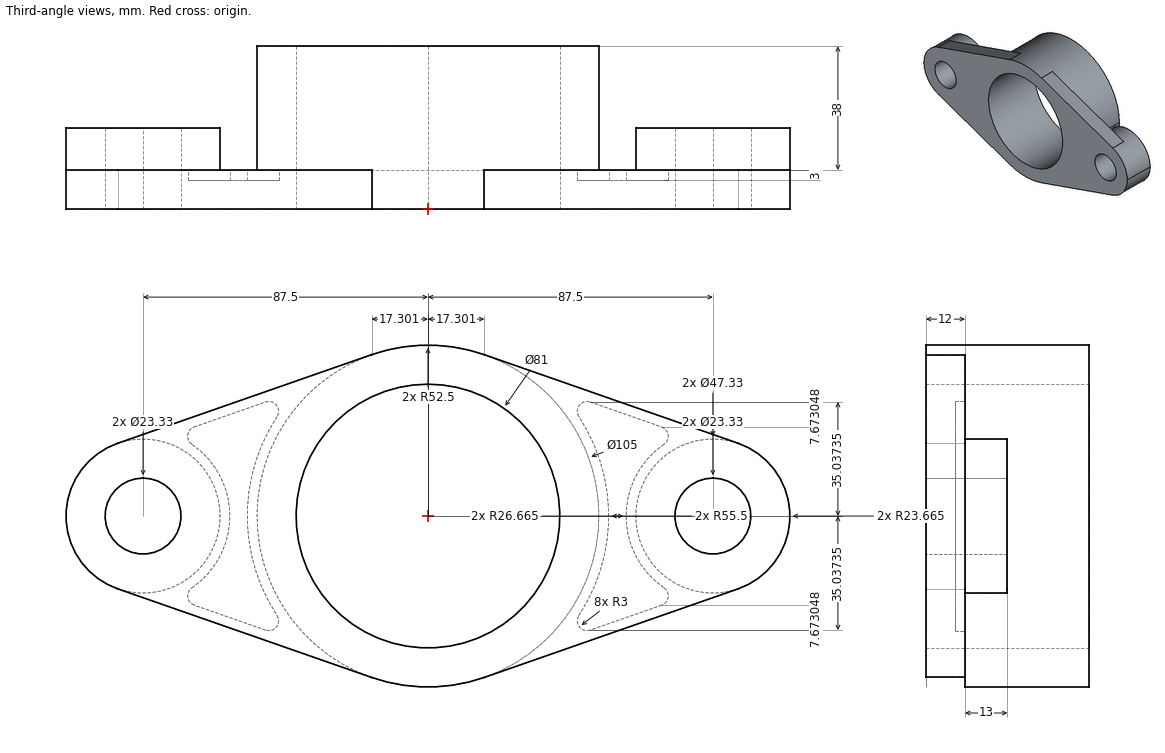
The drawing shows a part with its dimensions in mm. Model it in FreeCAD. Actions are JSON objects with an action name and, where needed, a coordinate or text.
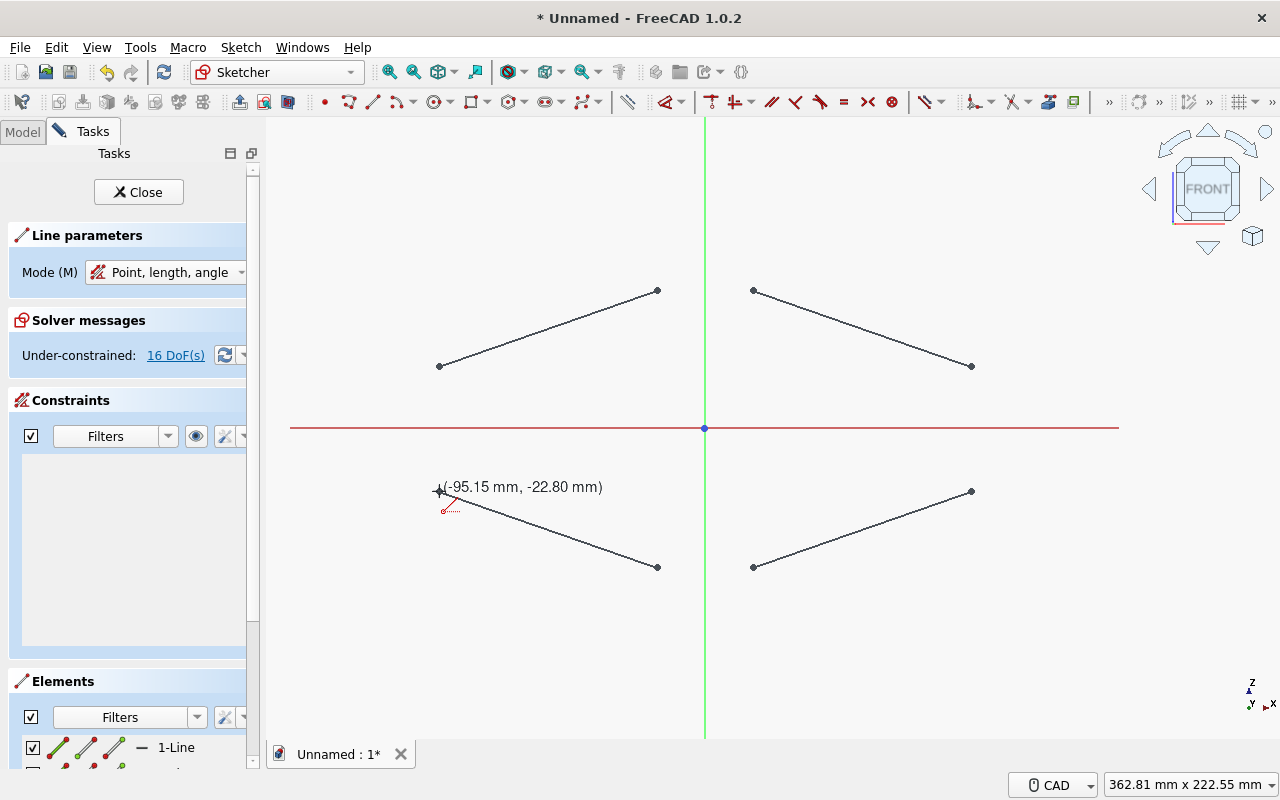
{"action": "key", "text": "g 3 a"}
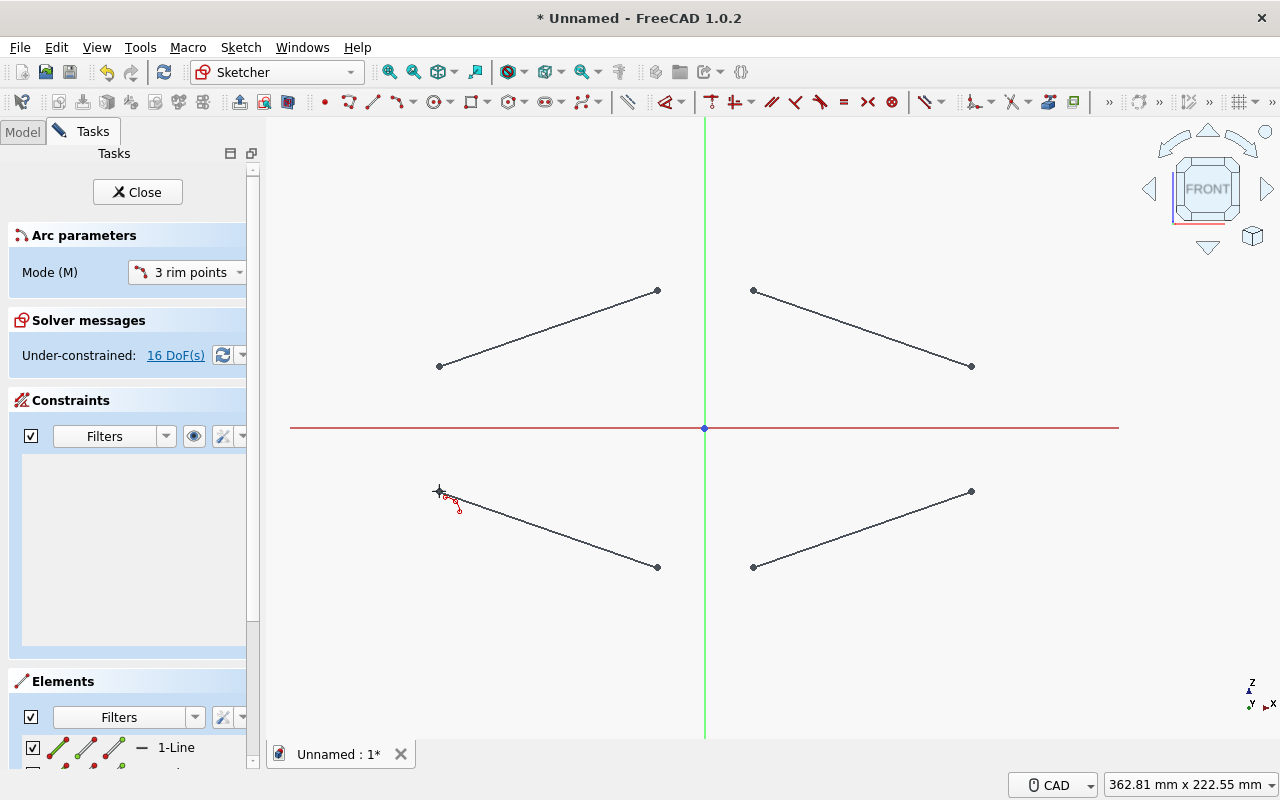
{"action": "left_click", "coordinate": [657, 291]}
{"action": "left_click", "coordinate": [753, 291]}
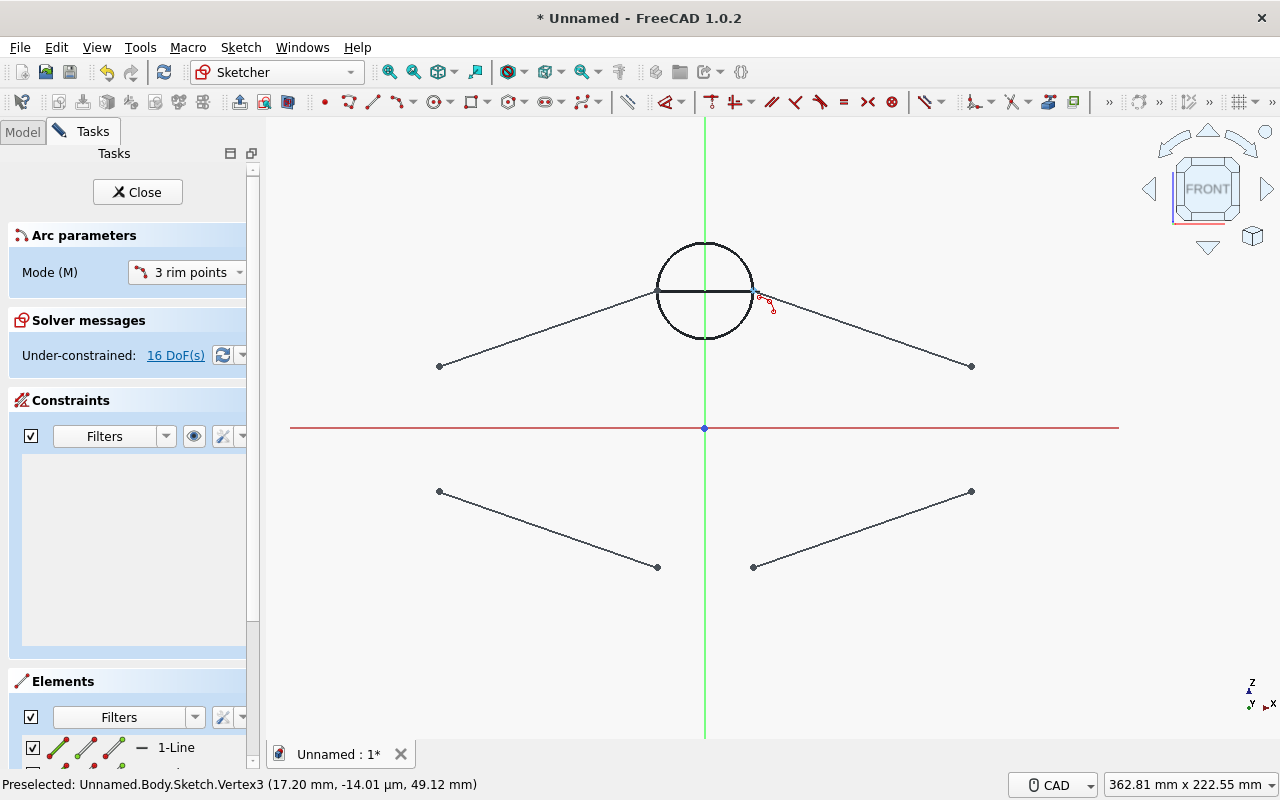
{"action": "scroll", "coordinate": [715, 282], "scroll_direction": "up", "scroll_amount": 4}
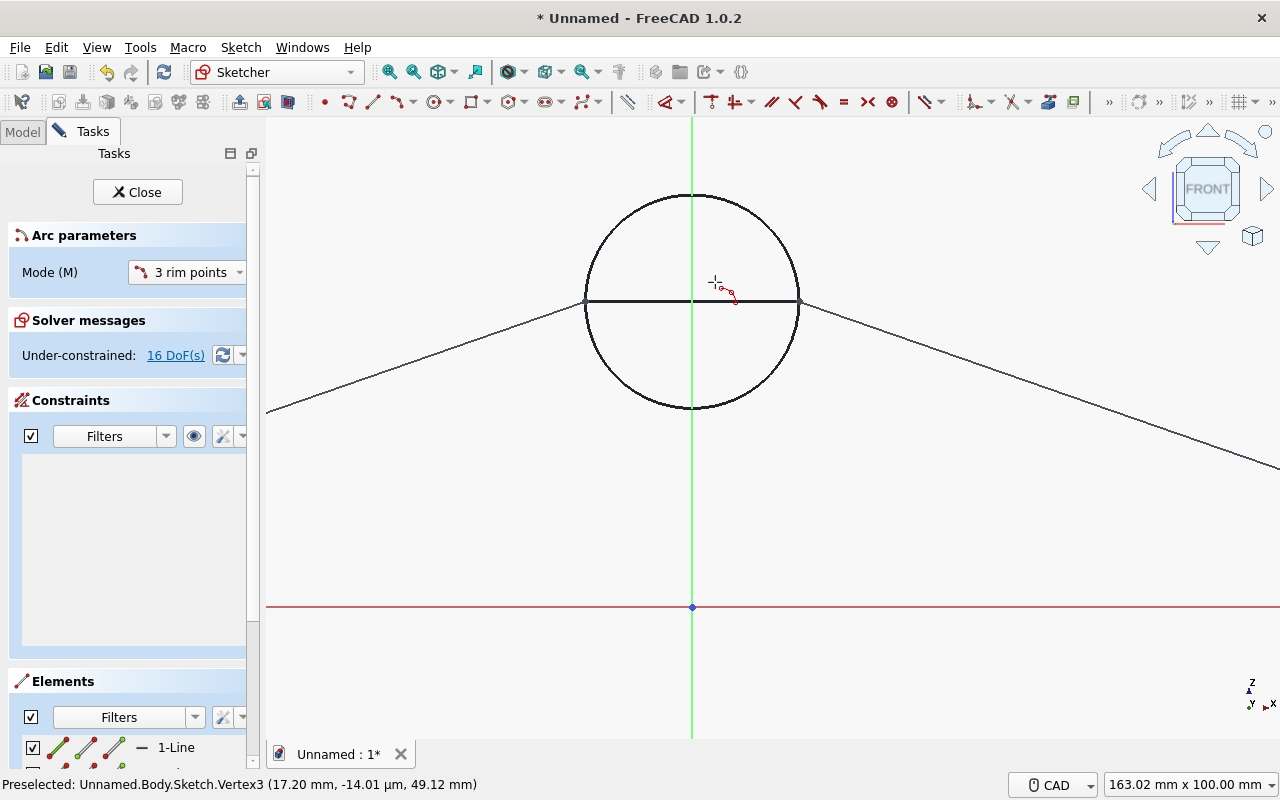
{"action": "left_click", "coordinate": [714, 281]}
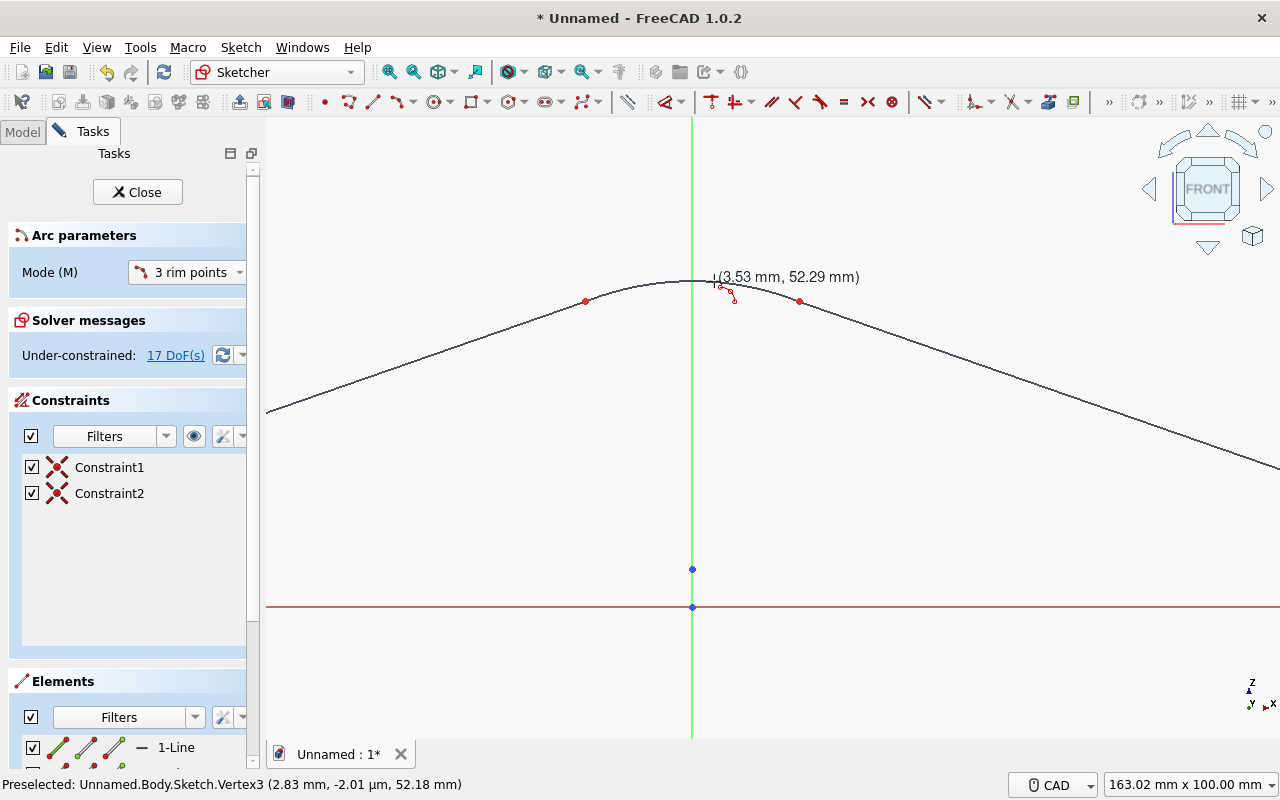
{"action": "scroll", "coordinate": [715, 282], "scroll_direction": "down", "scroll_amount": 4}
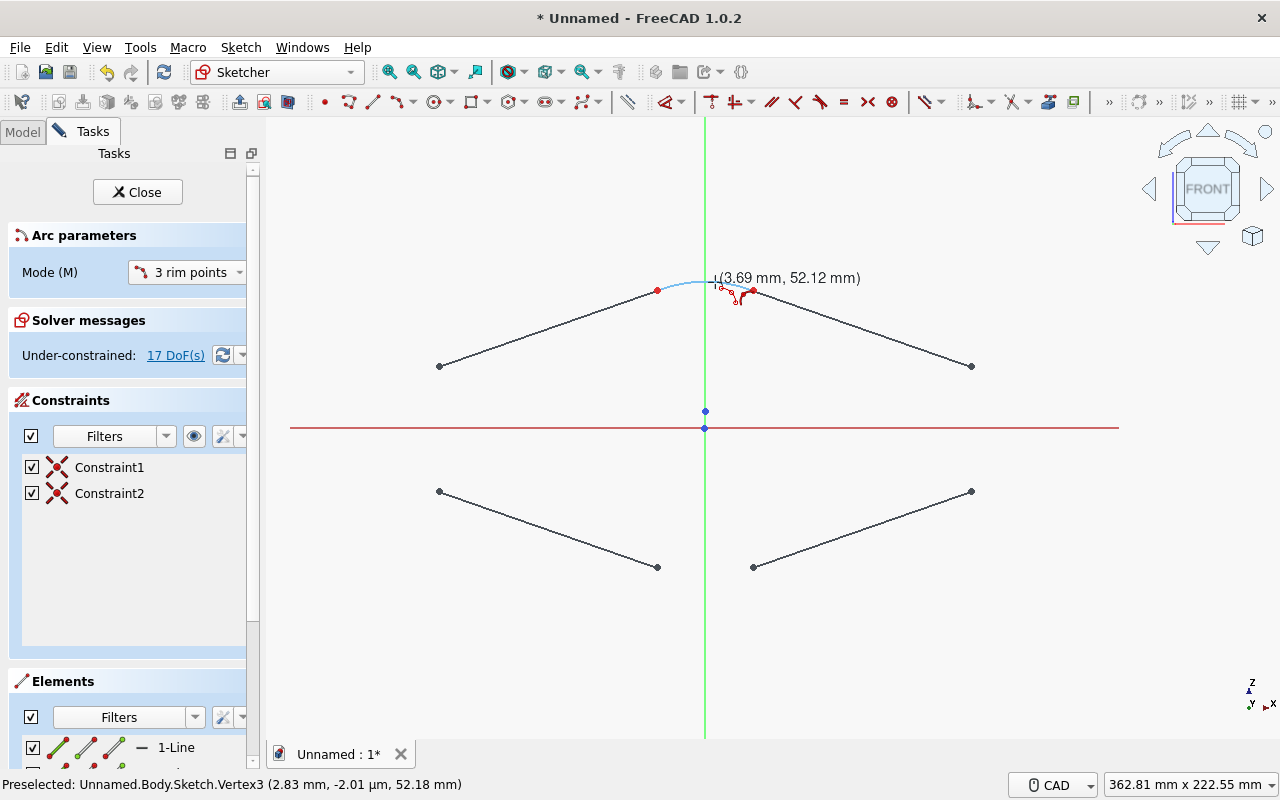
{"action": "left_click", "coordinate": [971, 367]}
{"action": "left_click", "coordinate": [971, 492]}
{"action": "left_click", "coordinate": [1014, 444]}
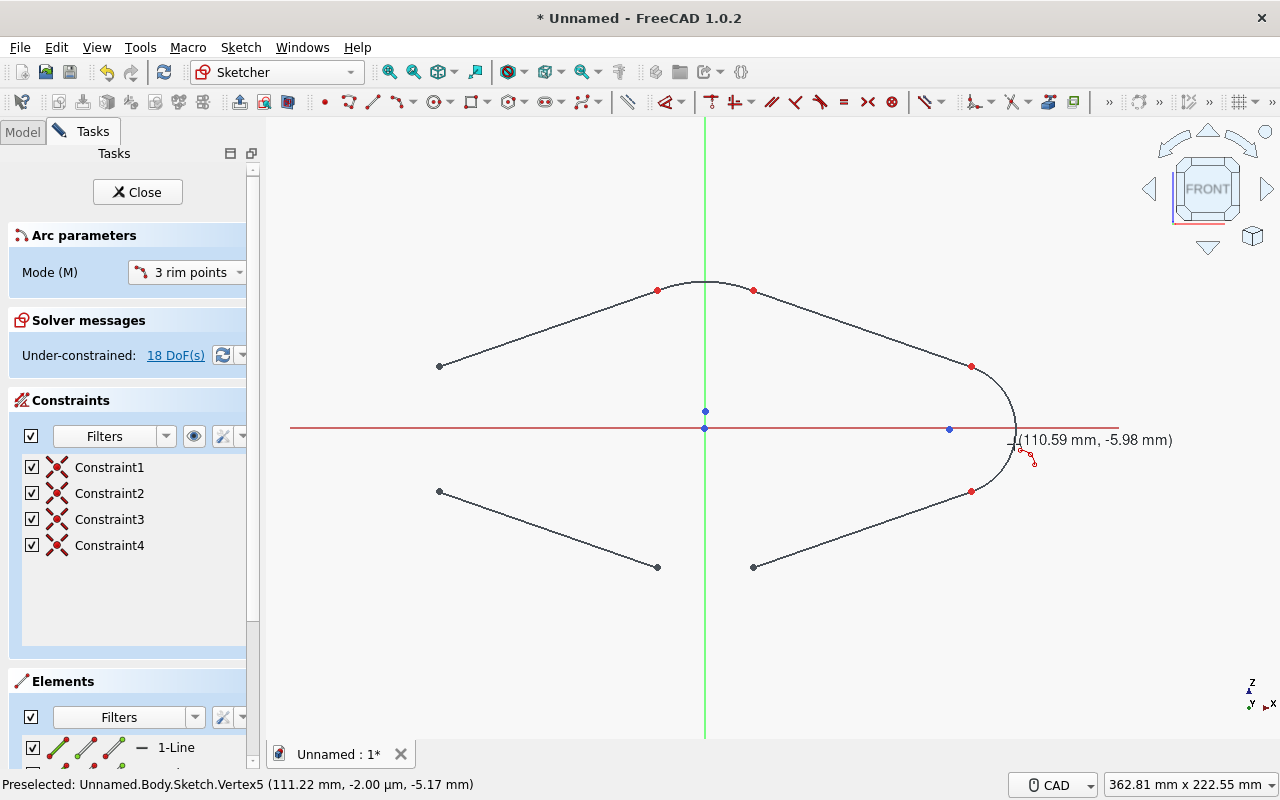
{"action": "left_click", "coordinate": [753, 568]}
{"action": "left_click", "coordinate": [657, 568]}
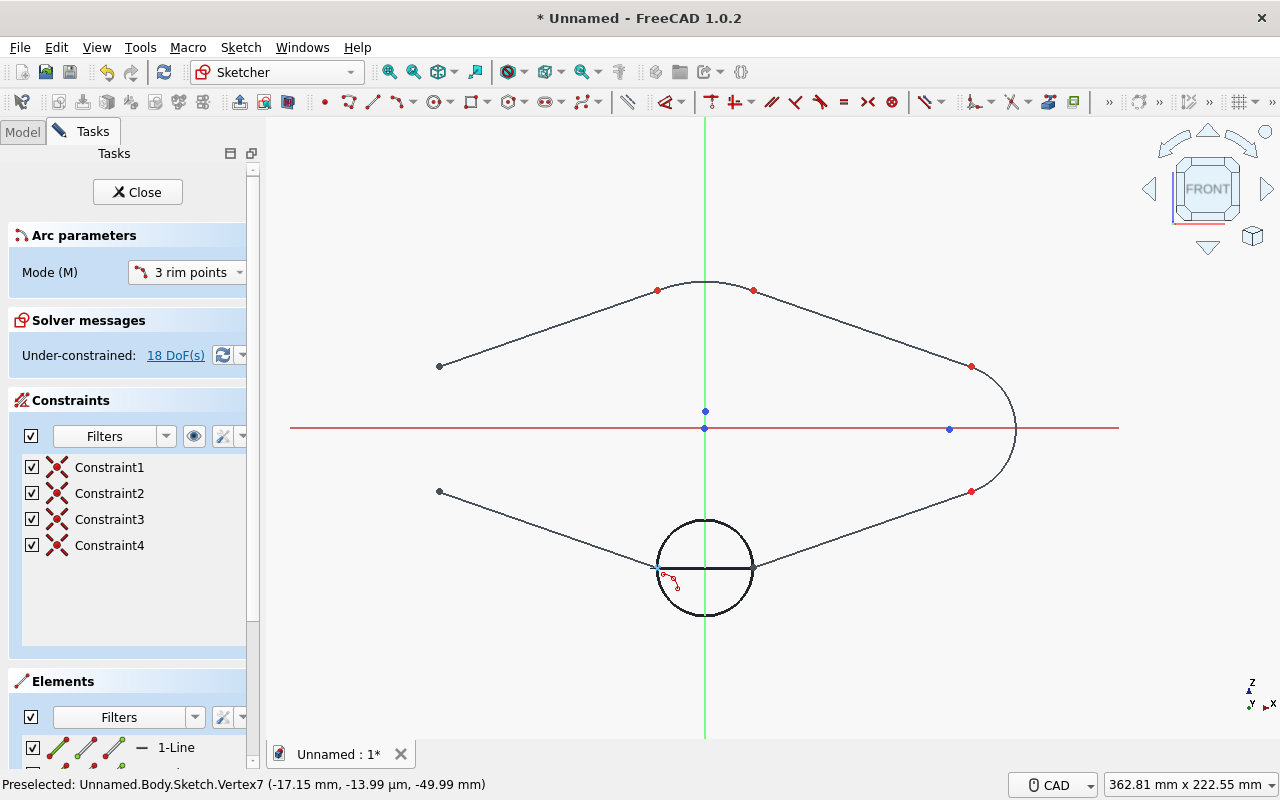
{"action": "scroll", "coordinate": [695, 575], "scroll_direction": "up", "scroll_amount": 4}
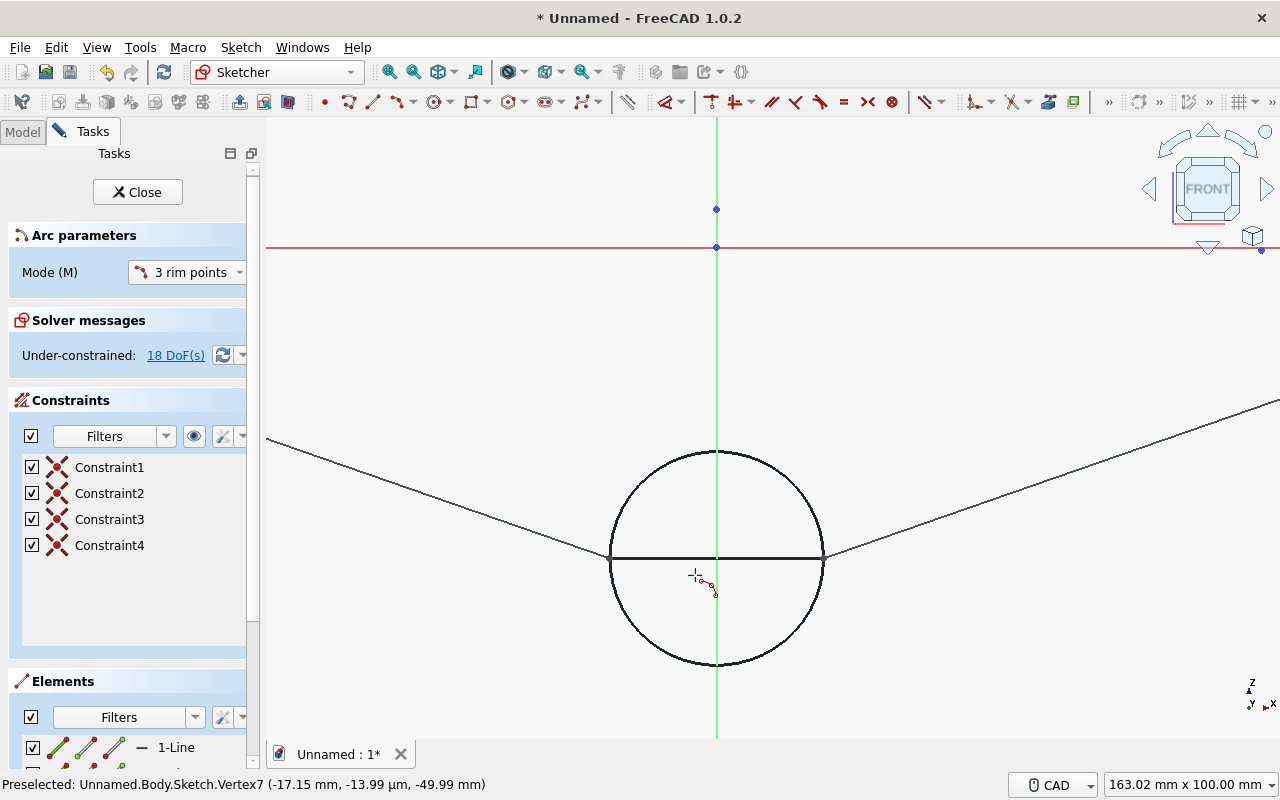
{"action": "left_click", "coordinate": [695, 573]}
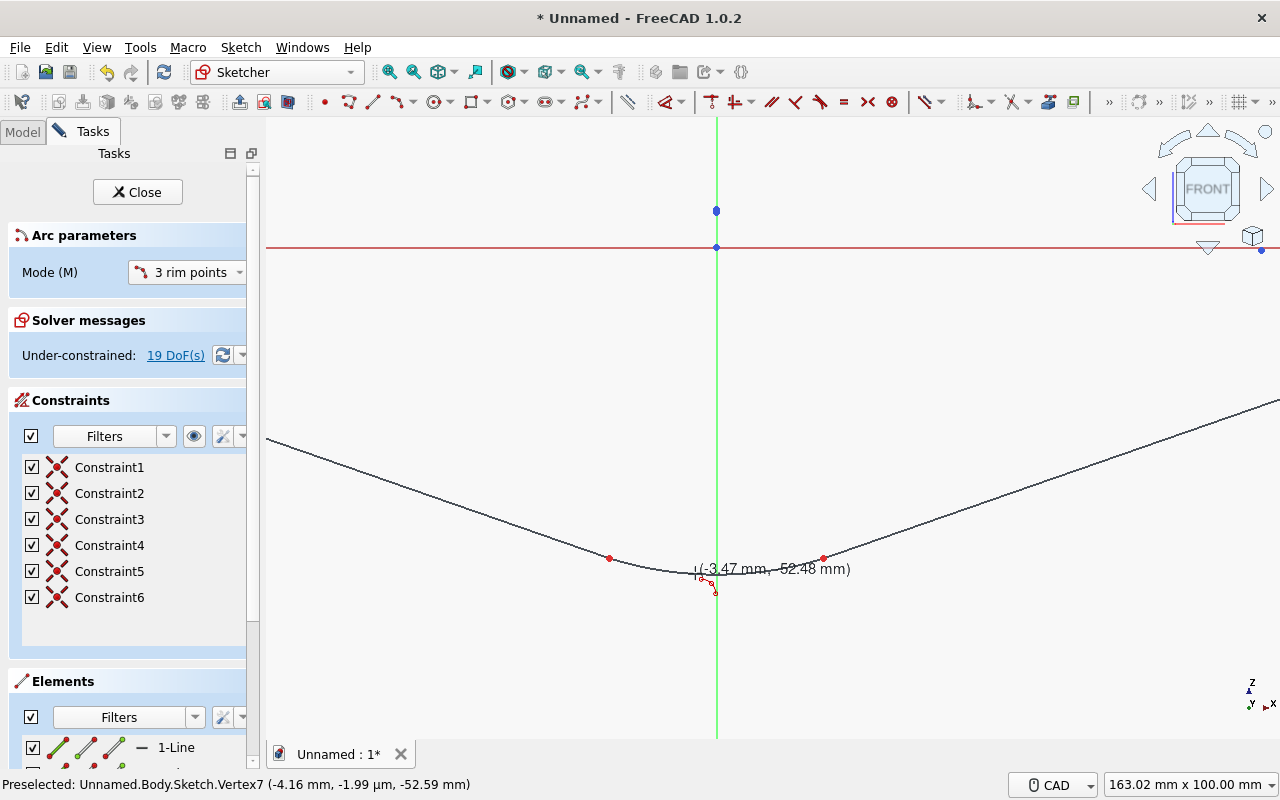
{"action": "scroll", "coordinate": [695, 575], "scroll_direction": "down", "scroll_amount": 4}